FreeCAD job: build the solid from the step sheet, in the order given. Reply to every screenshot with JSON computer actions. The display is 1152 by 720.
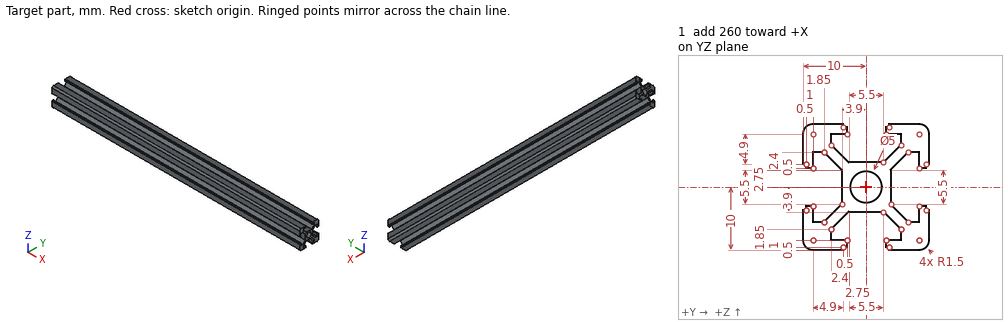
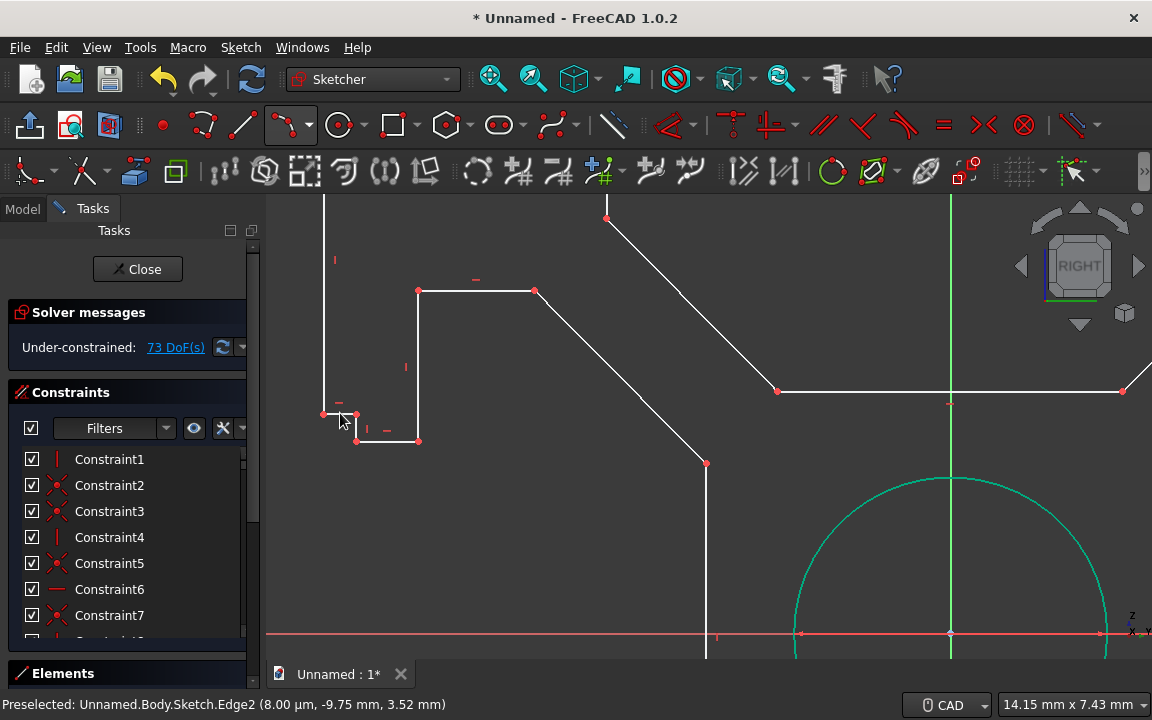
{"action": "scroll", "coordinate": [539, 359], "scroll_direction": "down", "scroll_amount": 7}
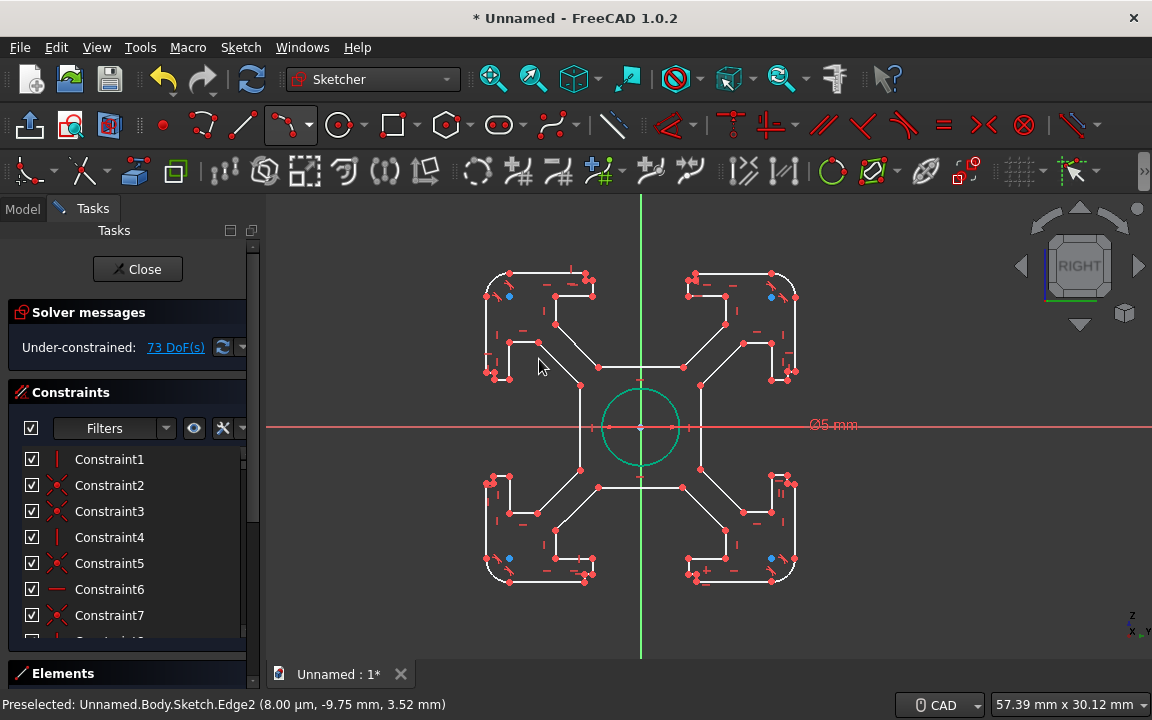
{"action": "scroll", "coordinate": [793, 484], "scroll_direction": "up", "scroll_amount": 10}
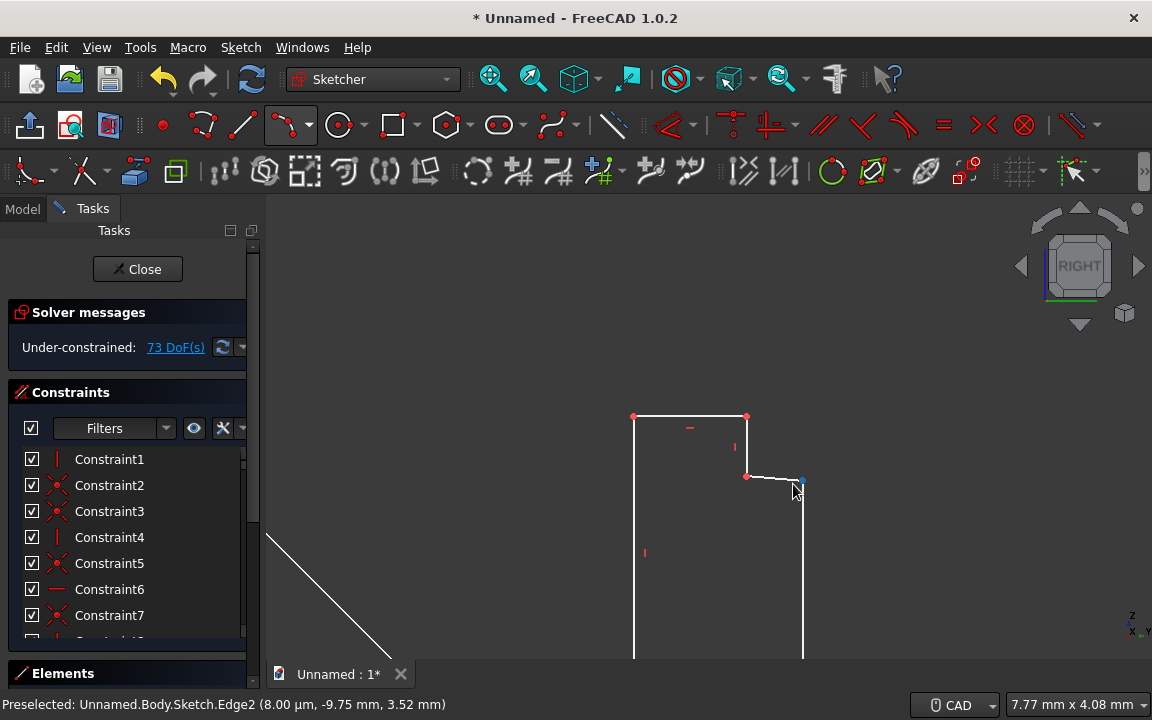
{"action": "left_click", "coordinate": [786, 479]}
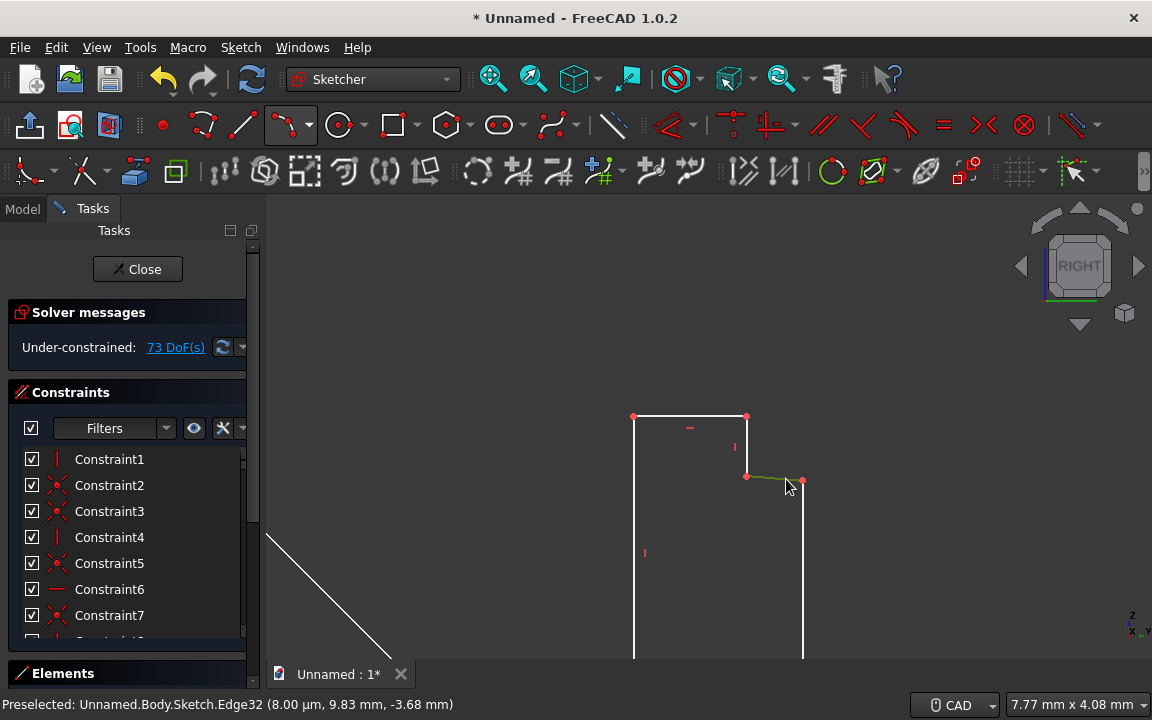
{"action": "key", "text": "h"}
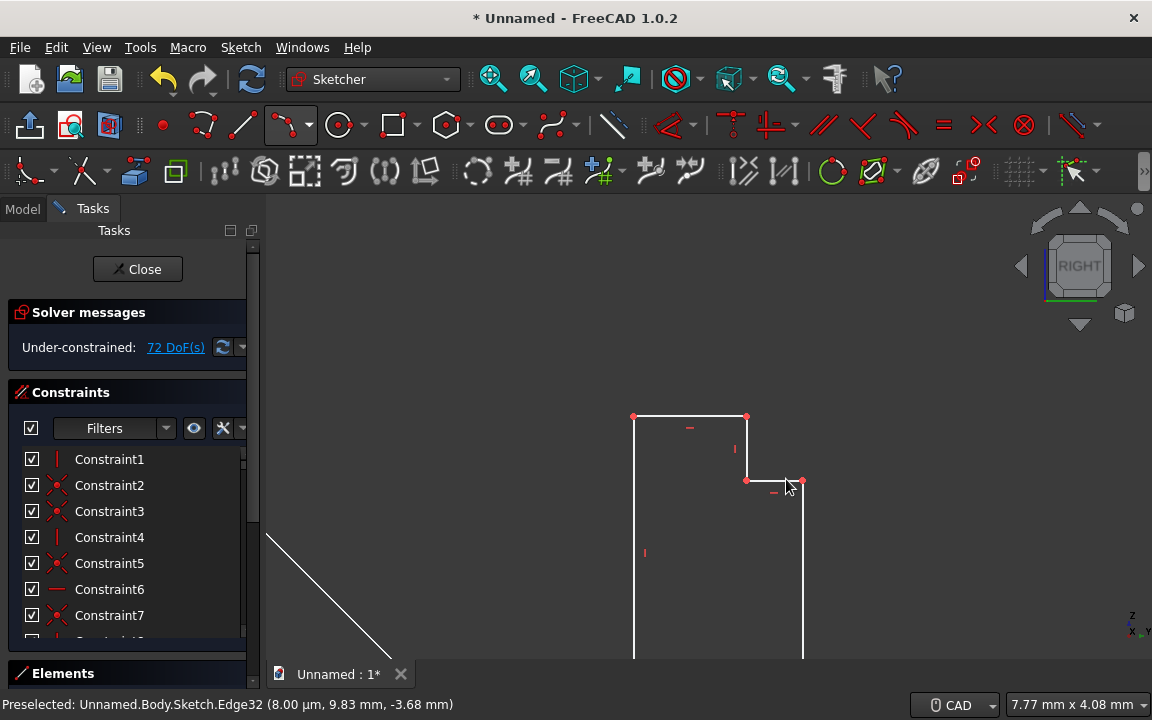
{"action": "scroll", "coordinate": [793, 484], "scroll_direction": "down", "scroll_amount": 10}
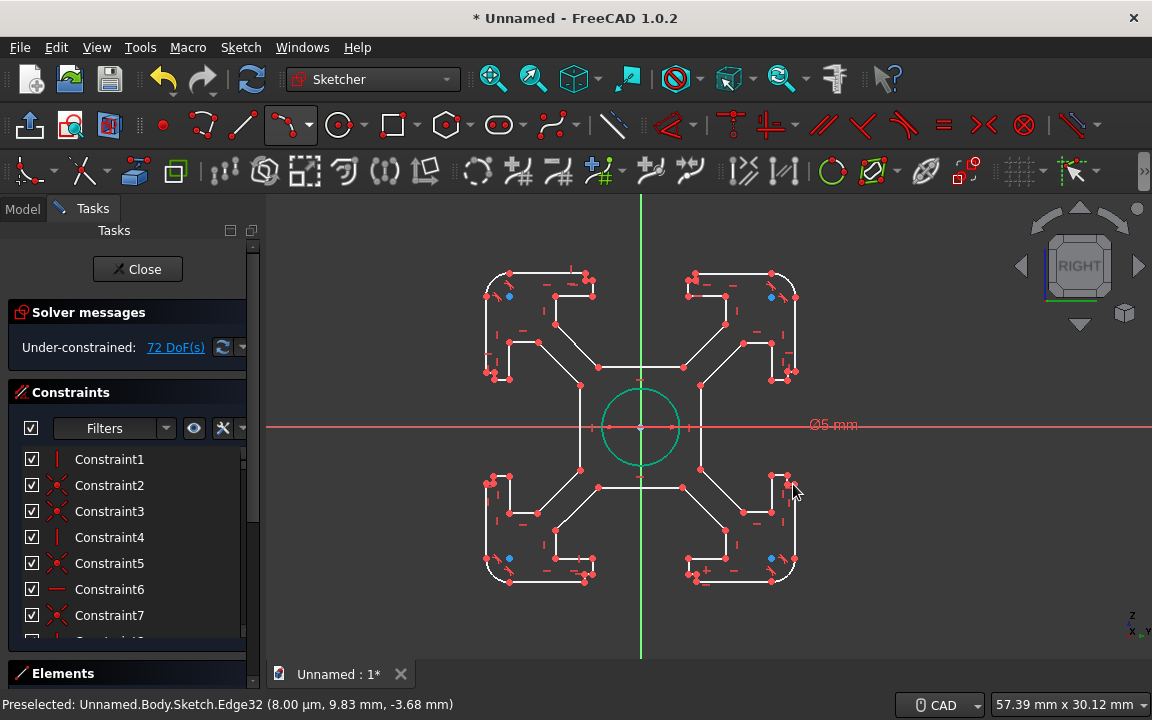
{"action": "scroll", "coordinate": [489, 570], "scroll_direction": "up", "scroll_amount": 2}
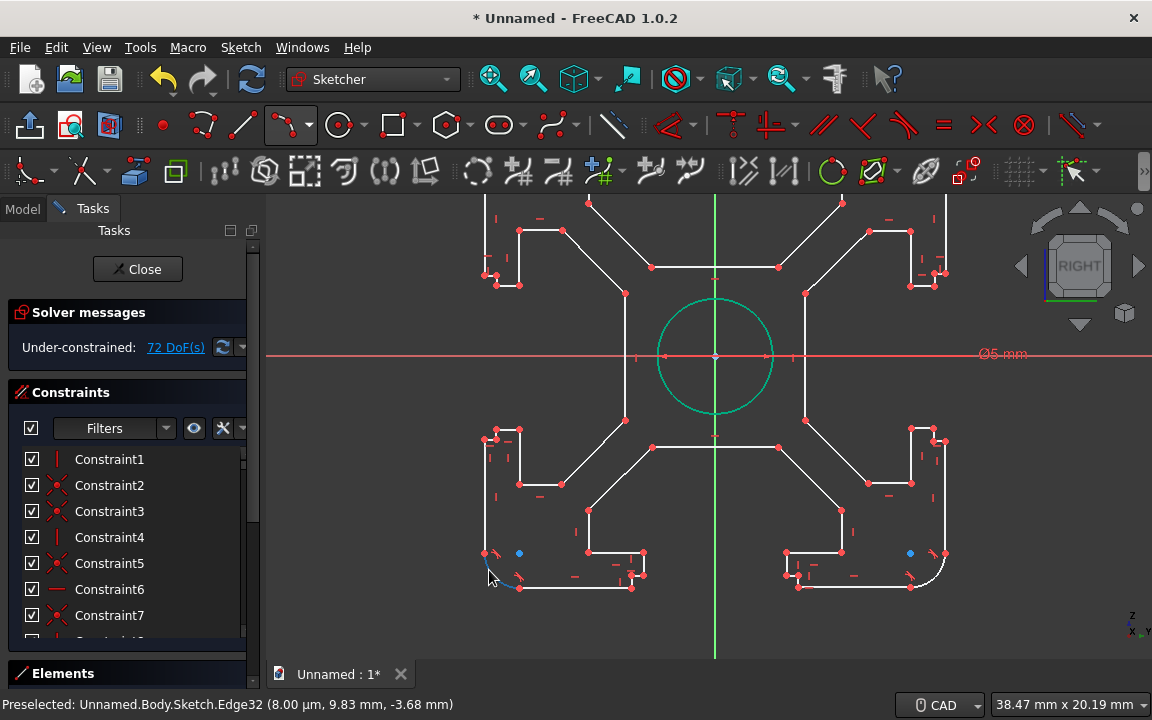
{"action": "left_click", "coordinate": [489, 569]}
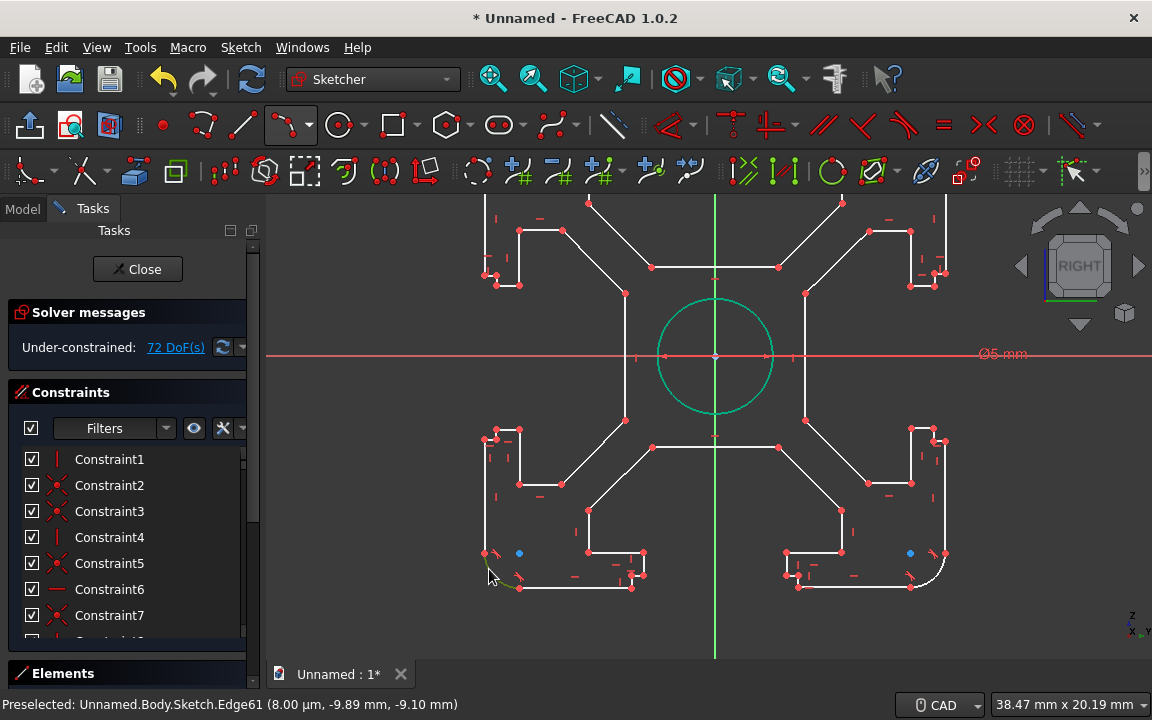
{"action": "left_click", "coordinate": [926, 584]}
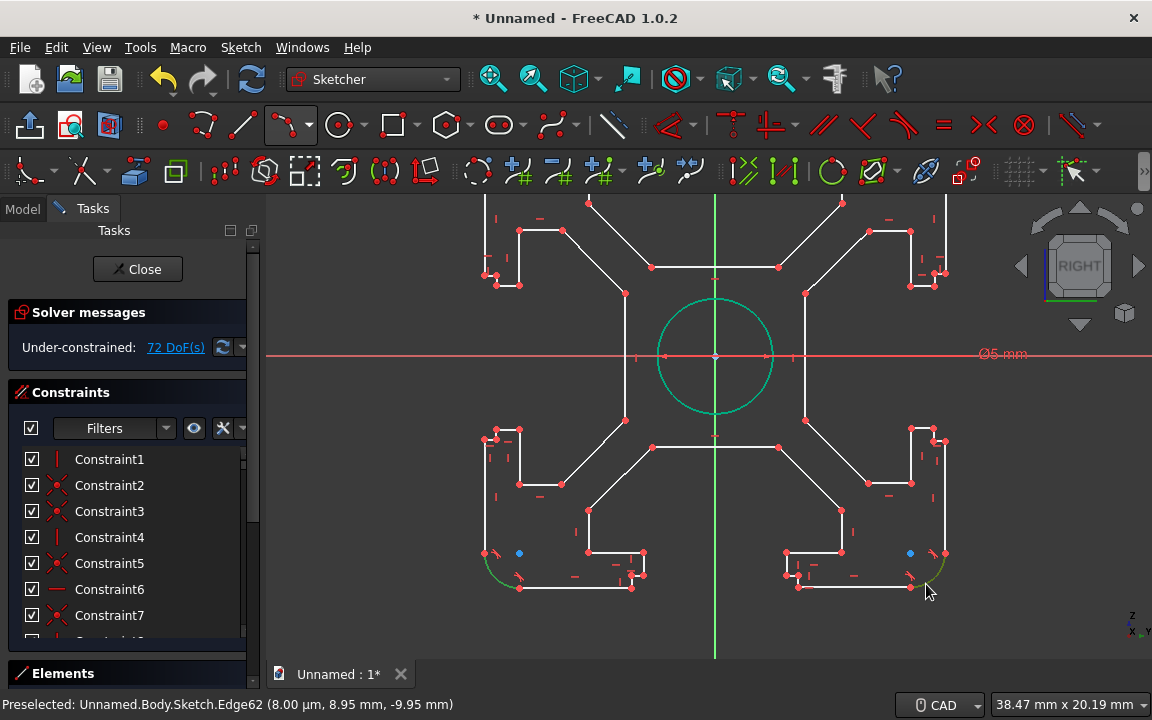
{"action": "scroll", "coordinate": [489, 569], "scroll_direction": "down", "scroll_amount": 2}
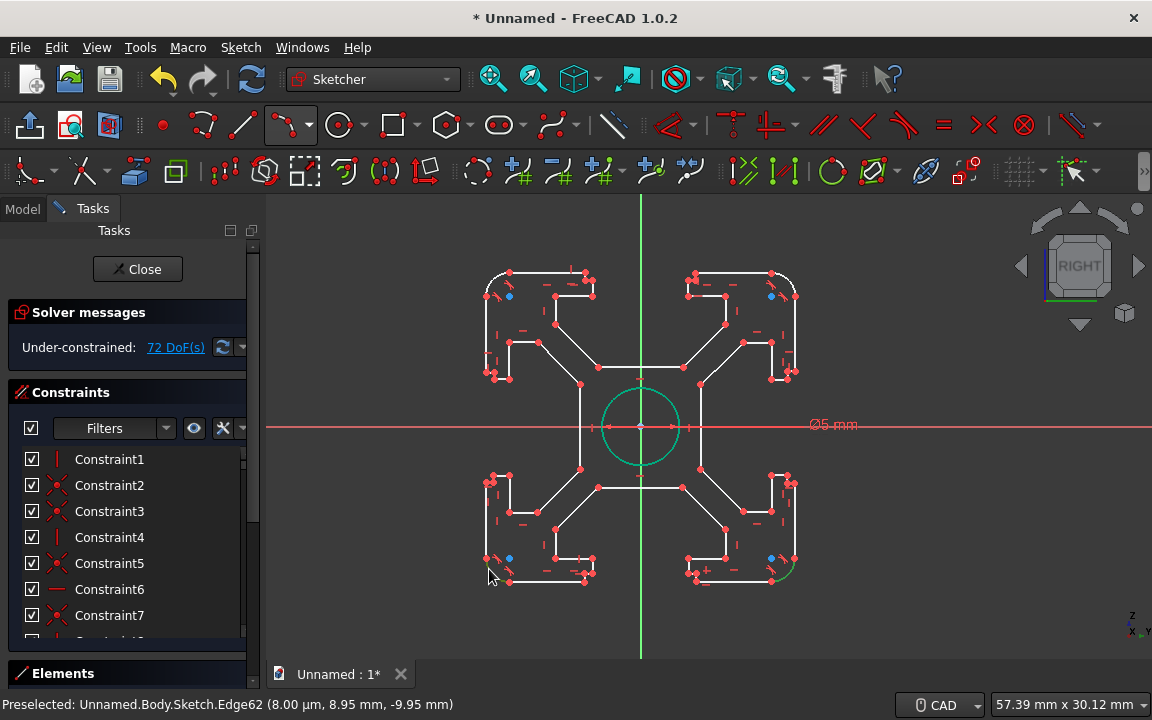
{"action": "scroll", "coordinate": [793, 286], "scroll_direction": "up", "scroll_amount": 2}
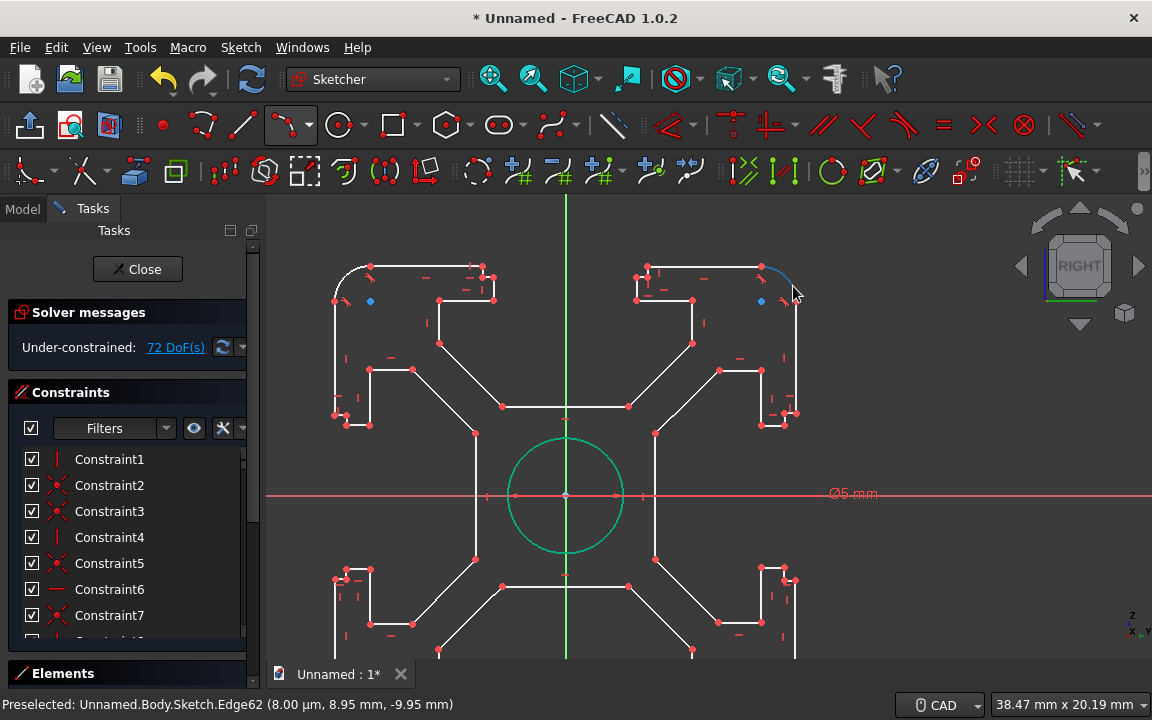
{"action": "left_click", "coordinate": [792, 286]}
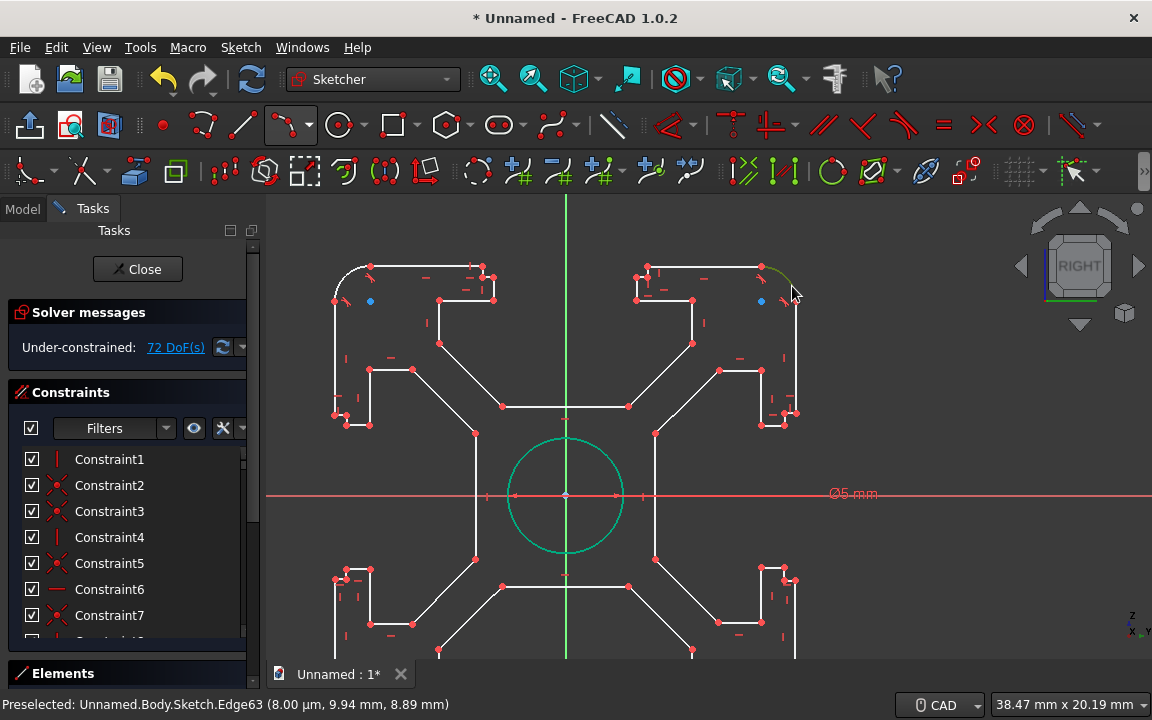
{"action": "left_click", "coordinate": [354, 270]}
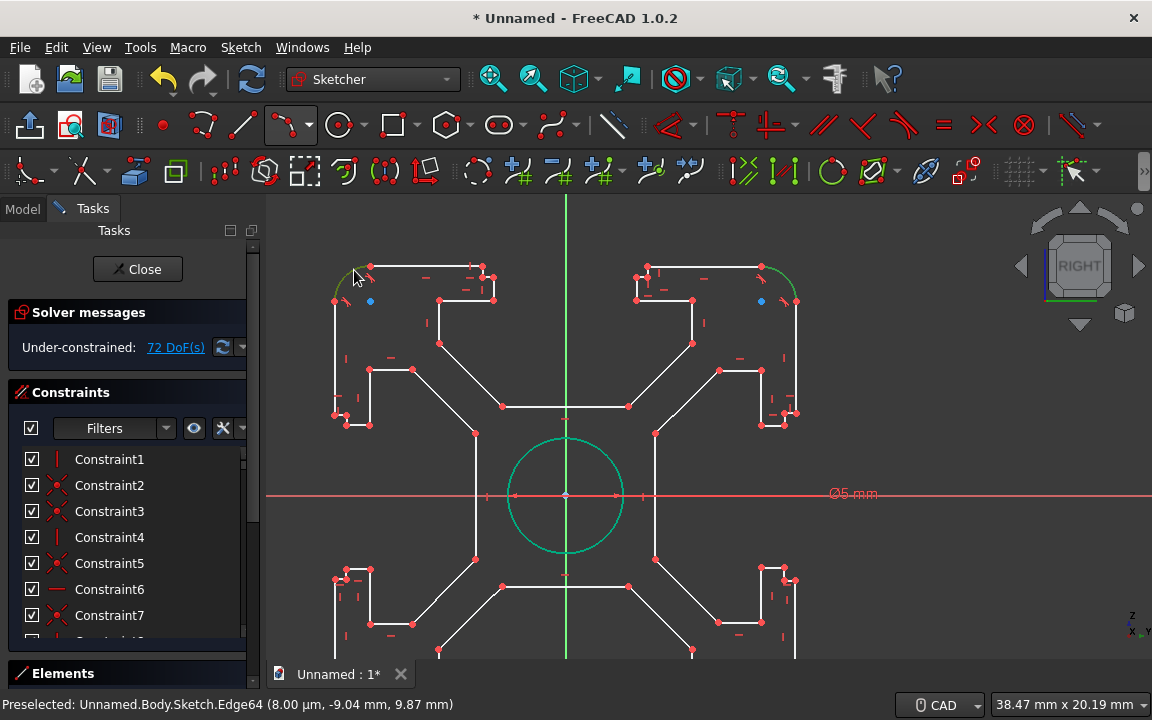
{"action": "key", "text": "e"}